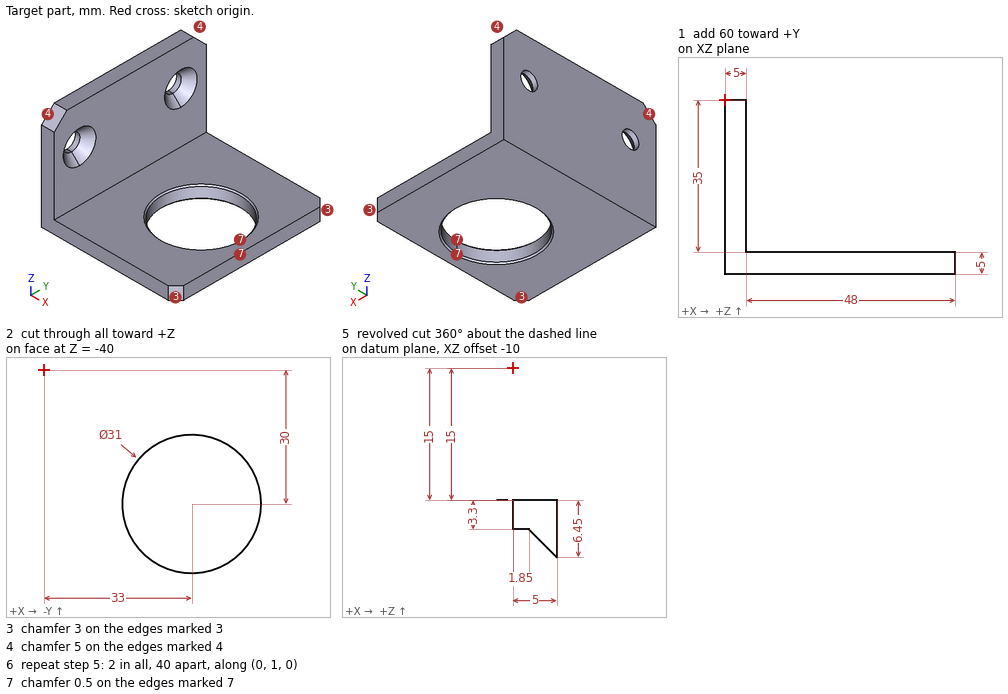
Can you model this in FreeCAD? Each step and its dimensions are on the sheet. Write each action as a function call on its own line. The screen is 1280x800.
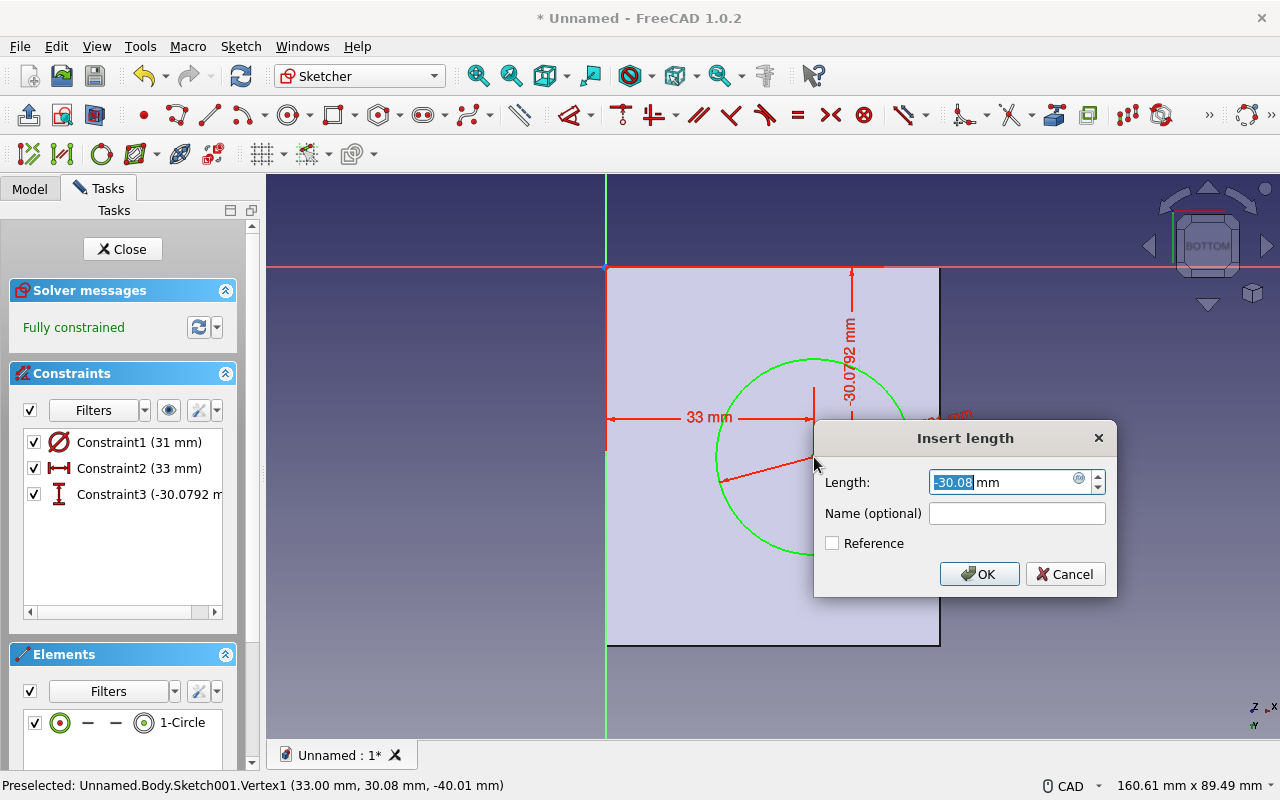
text(-30)
key(Return)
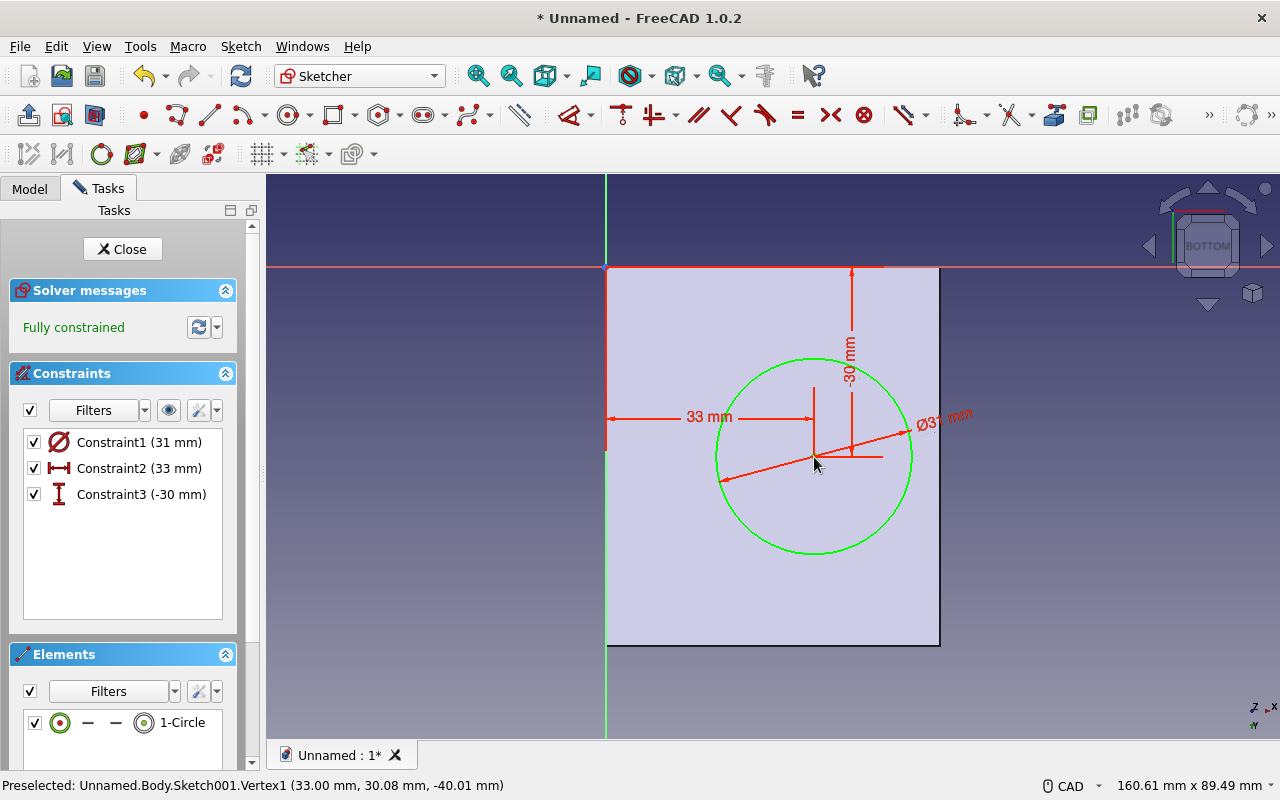
click(123, 249)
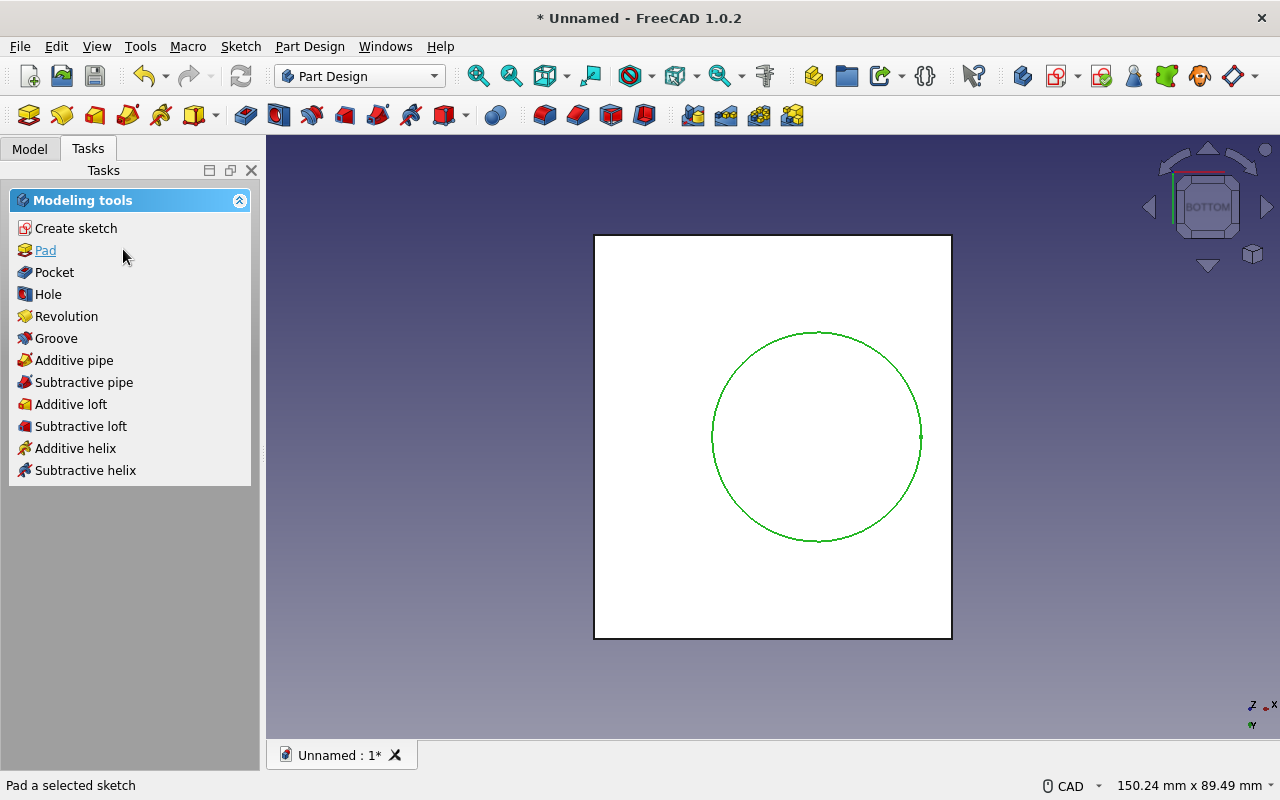
click(246, 116)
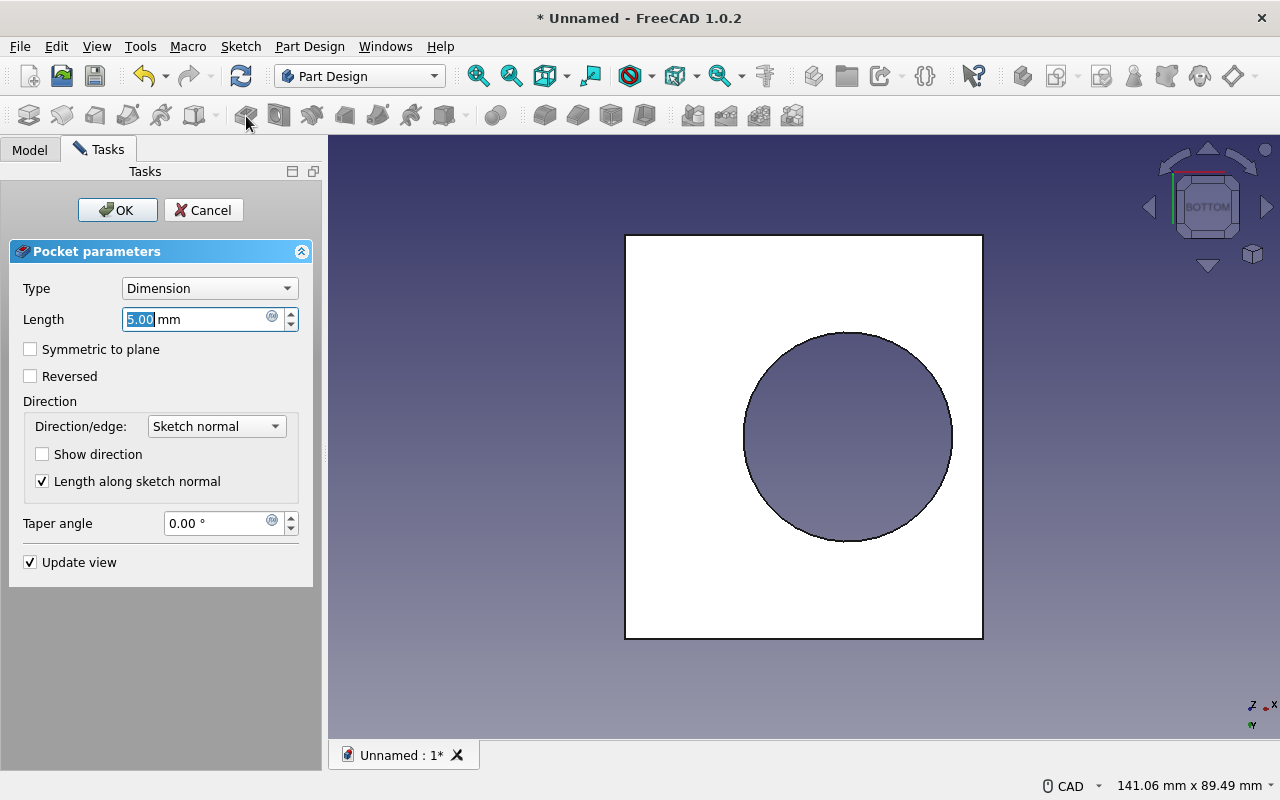
click(210, 288)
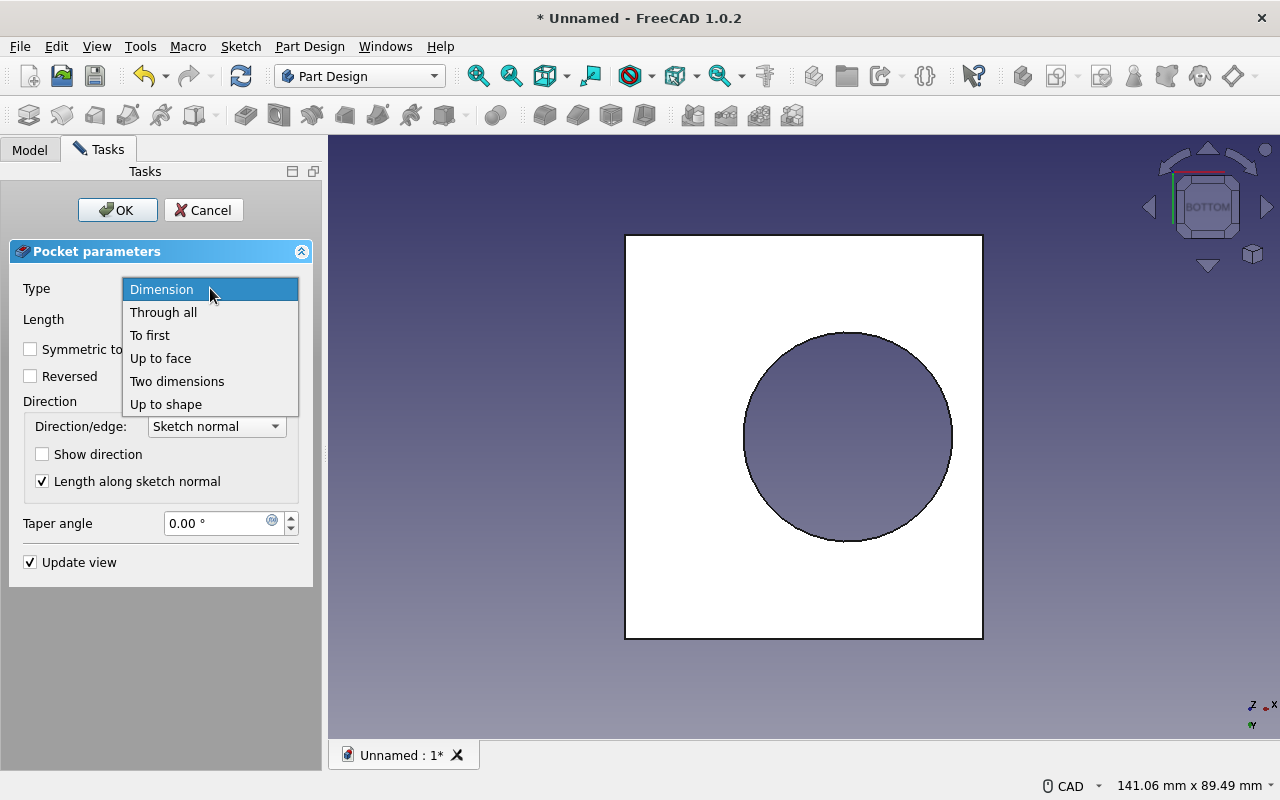
click(208, 312)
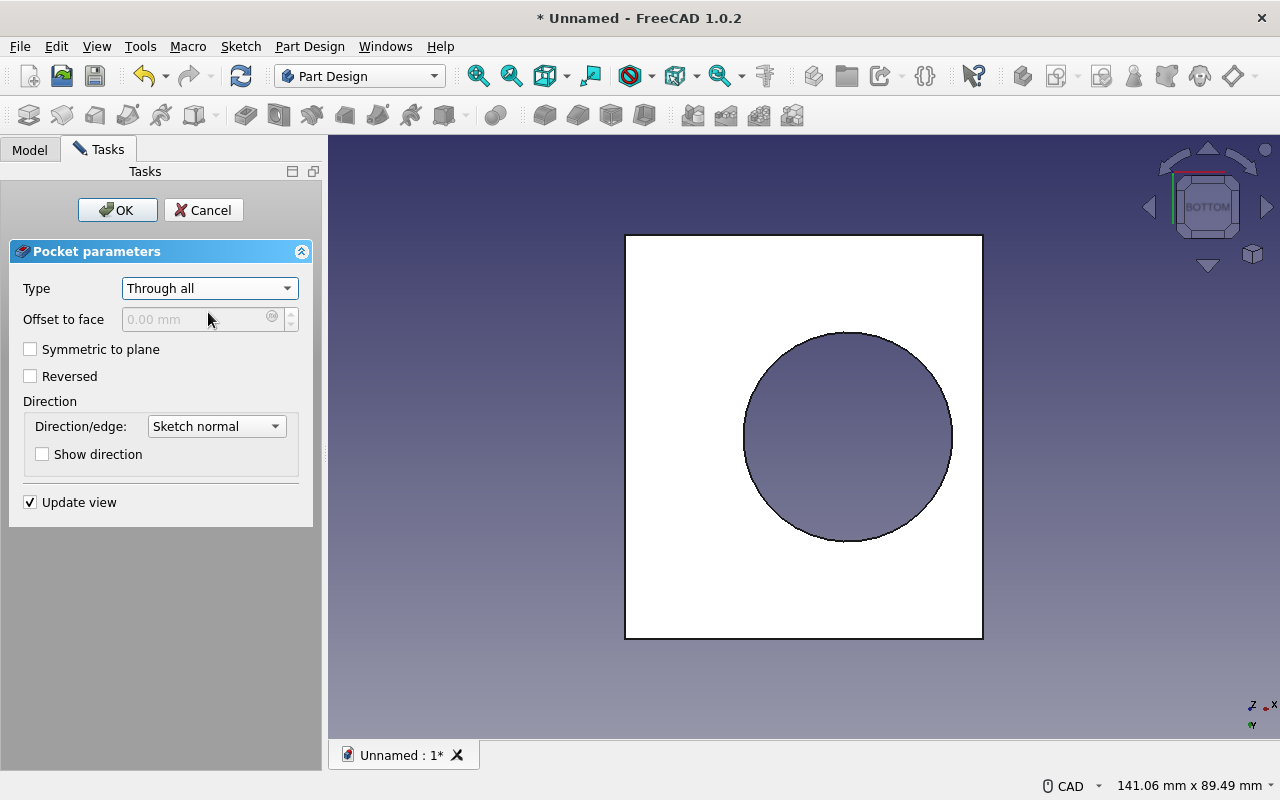
click(118, 210)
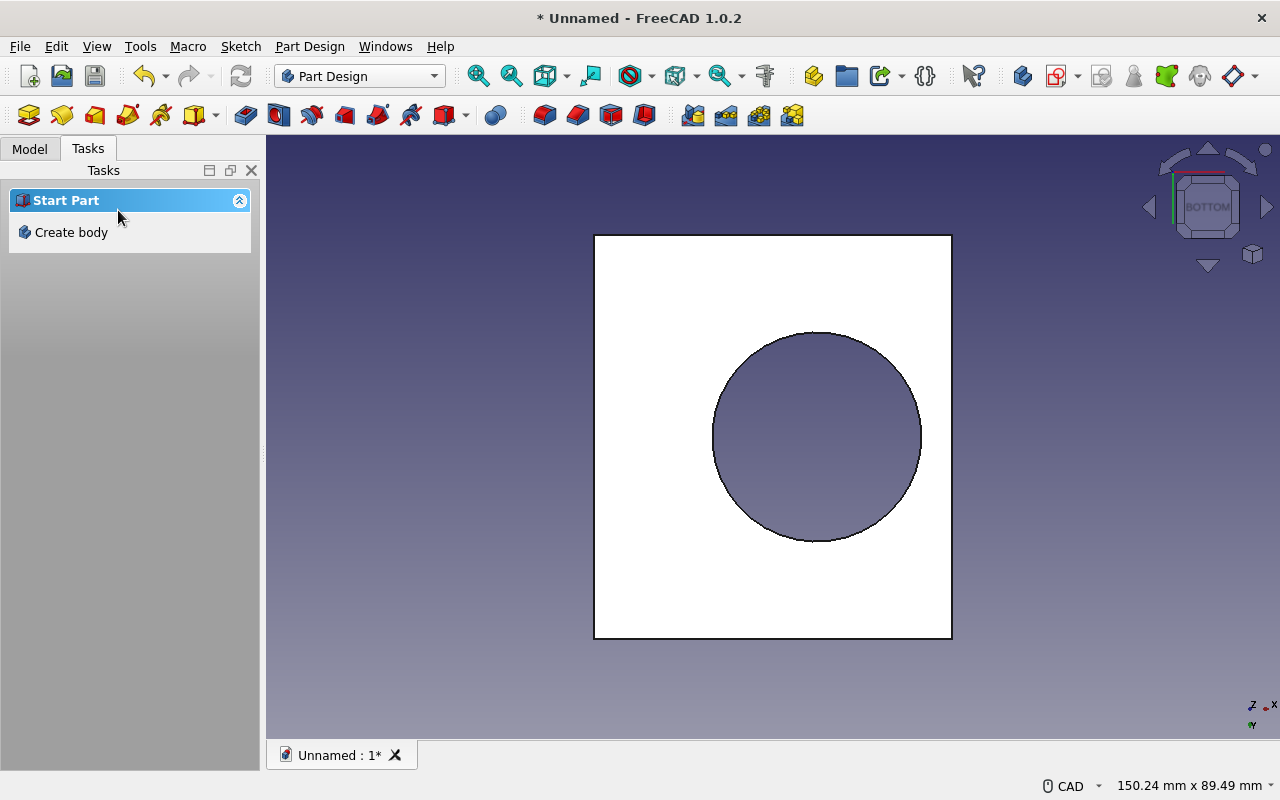
key(0)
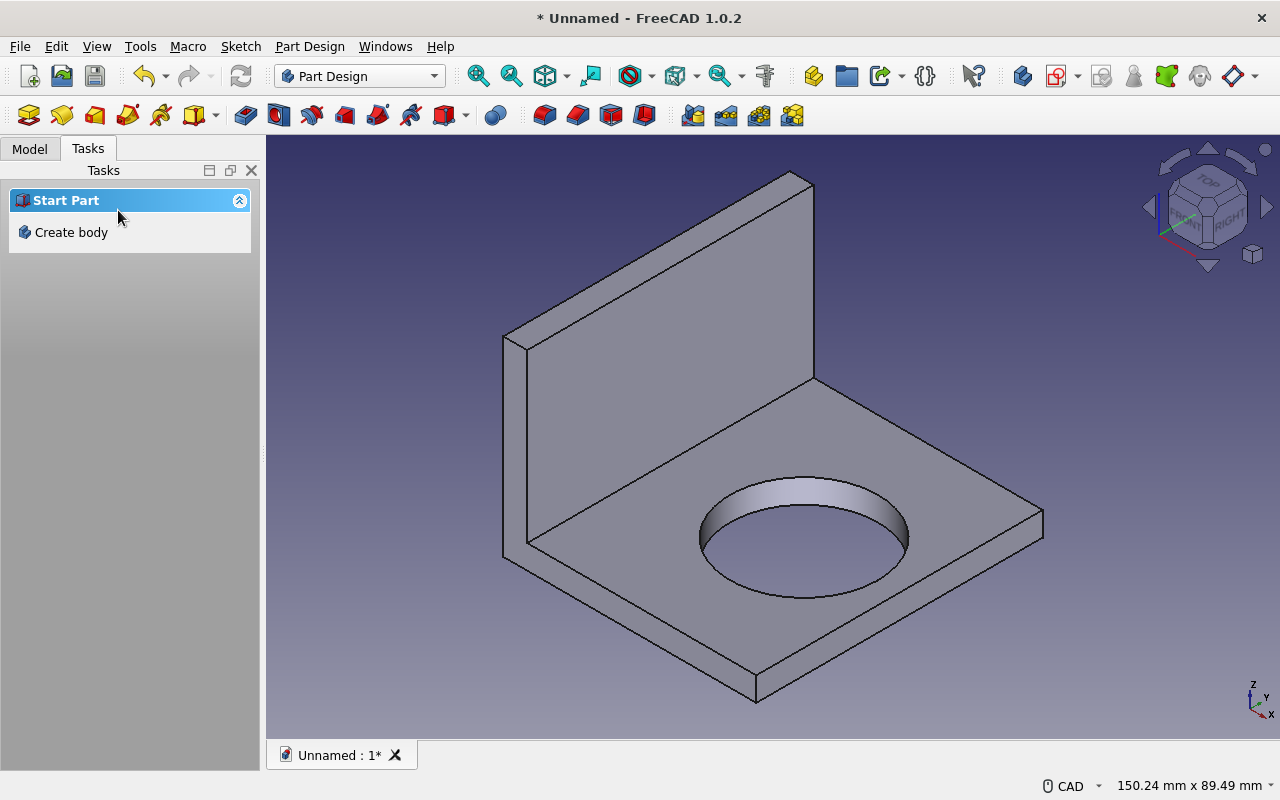
click(756, 688)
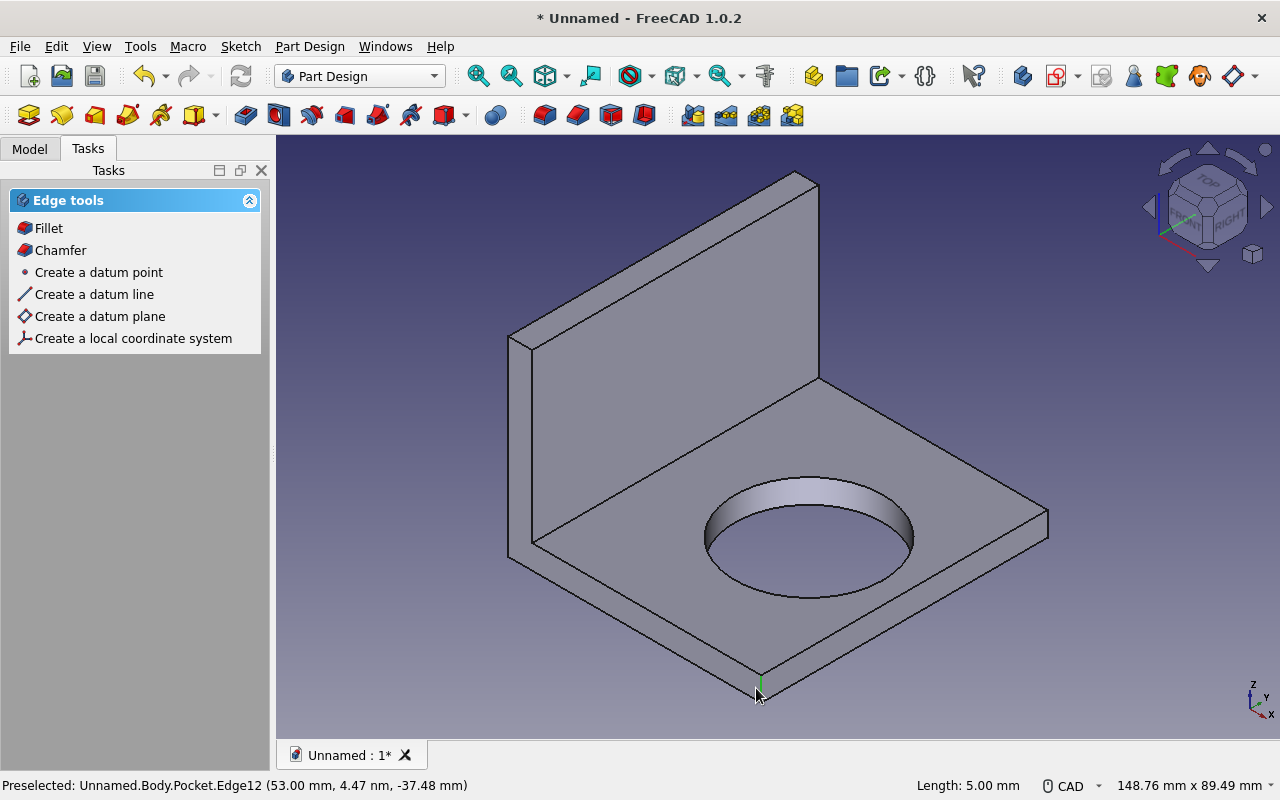
key(2)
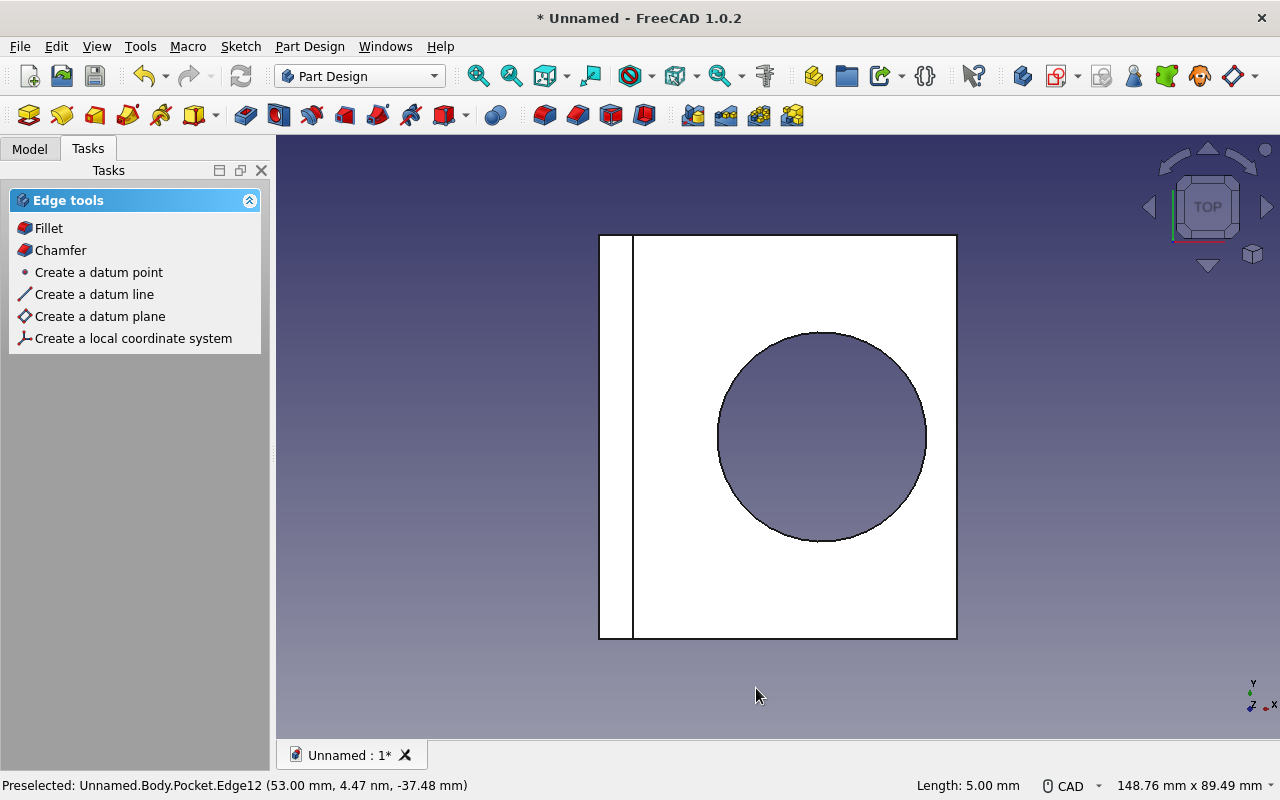
key(1)